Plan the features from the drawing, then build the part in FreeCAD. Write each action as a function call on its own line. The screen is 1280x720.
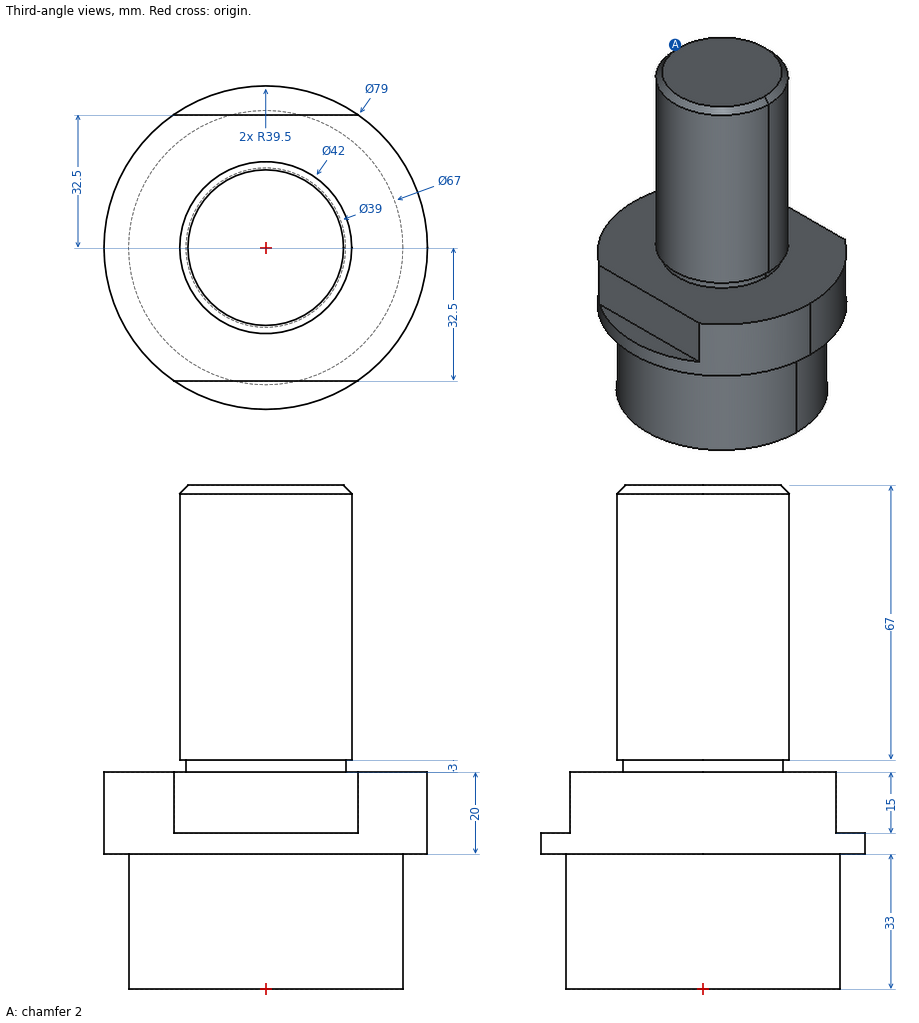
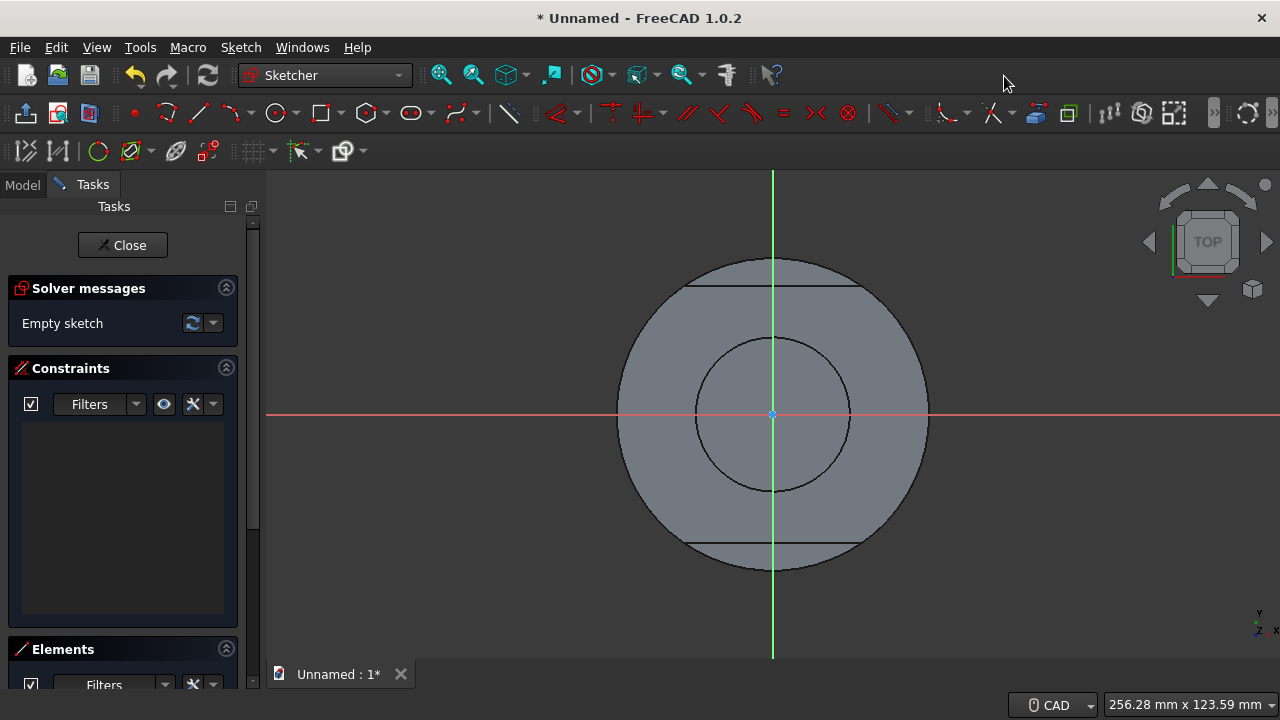
scroll(856, 415, up, 3)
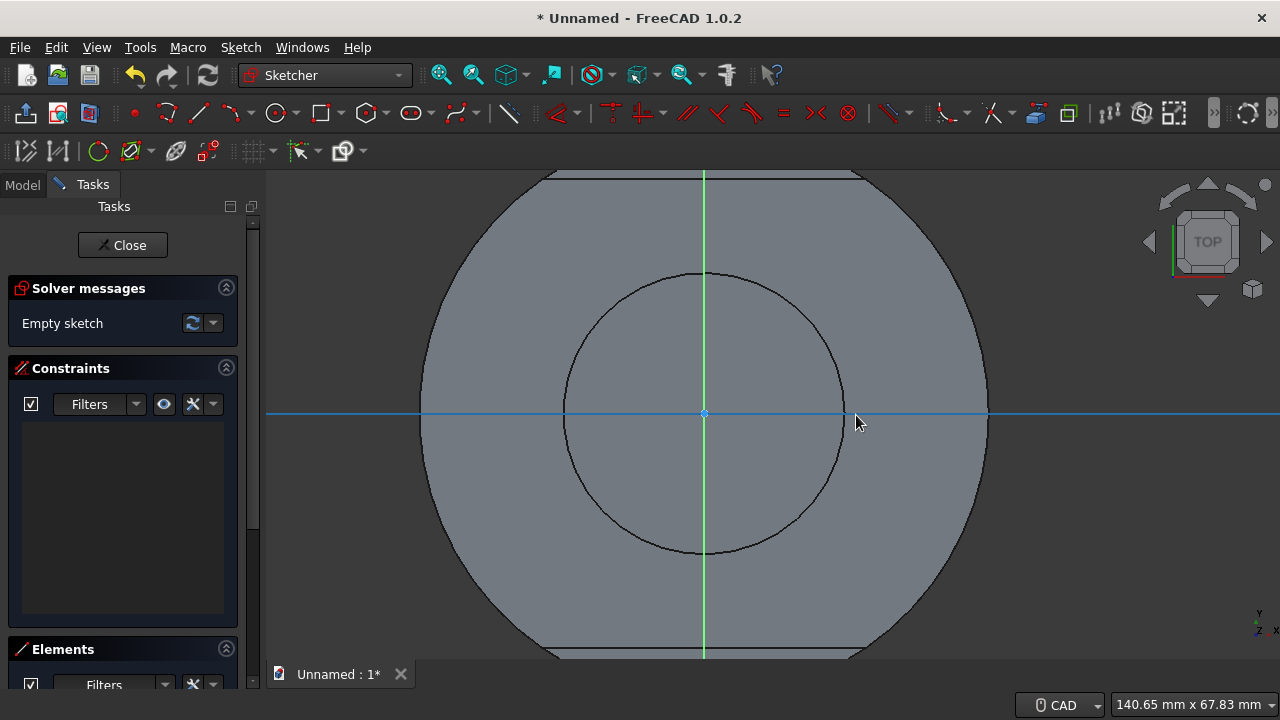
click(276, 114)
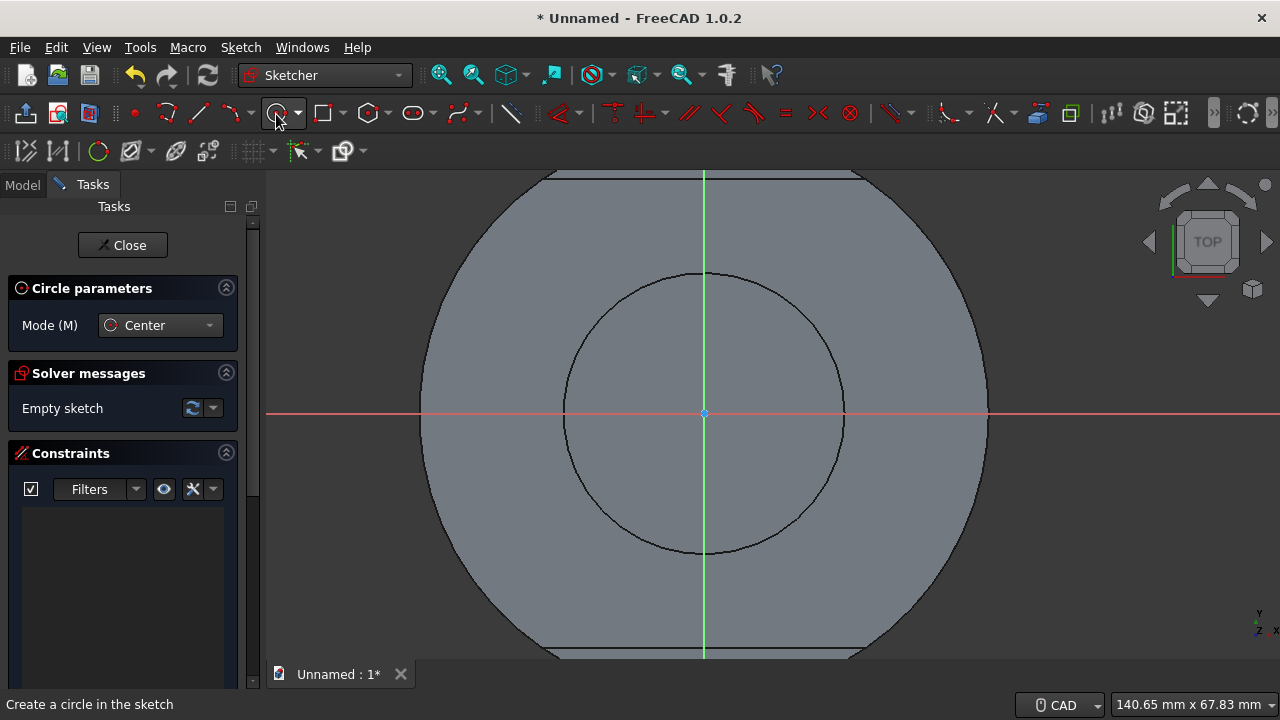
click(704, 414)
move(811, 307)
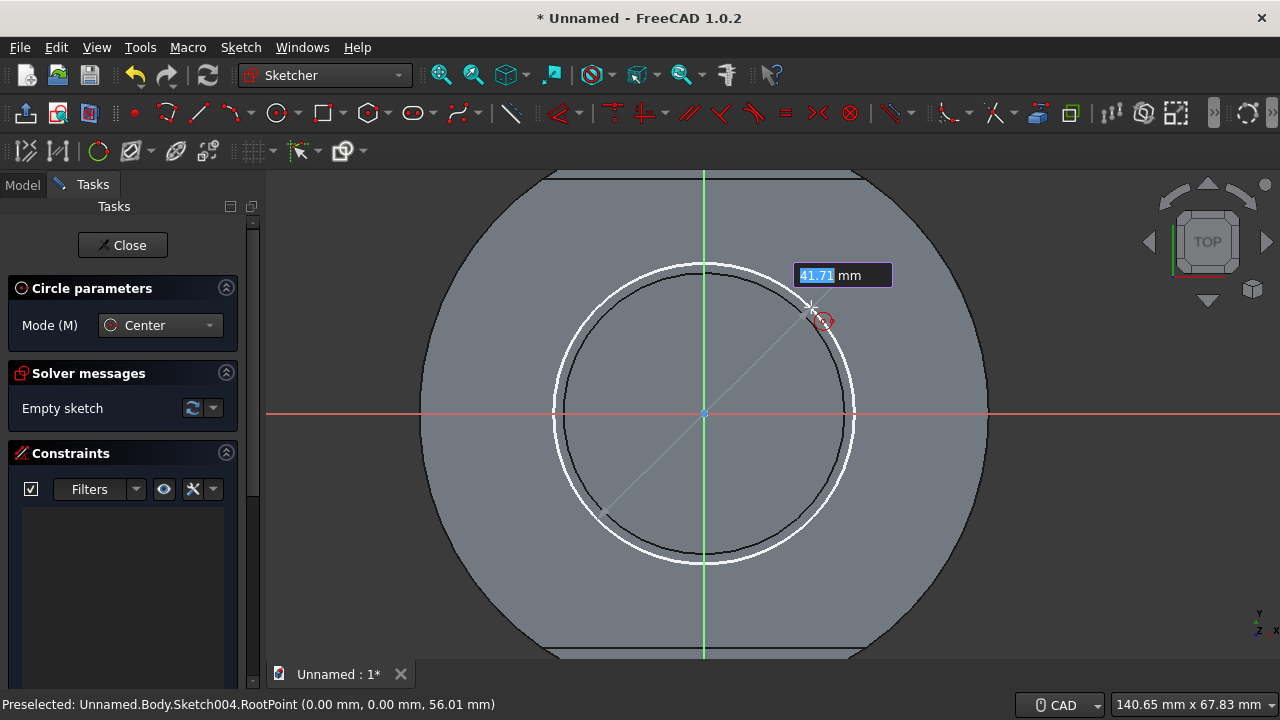
text(42)
key(Return)
key(Escape)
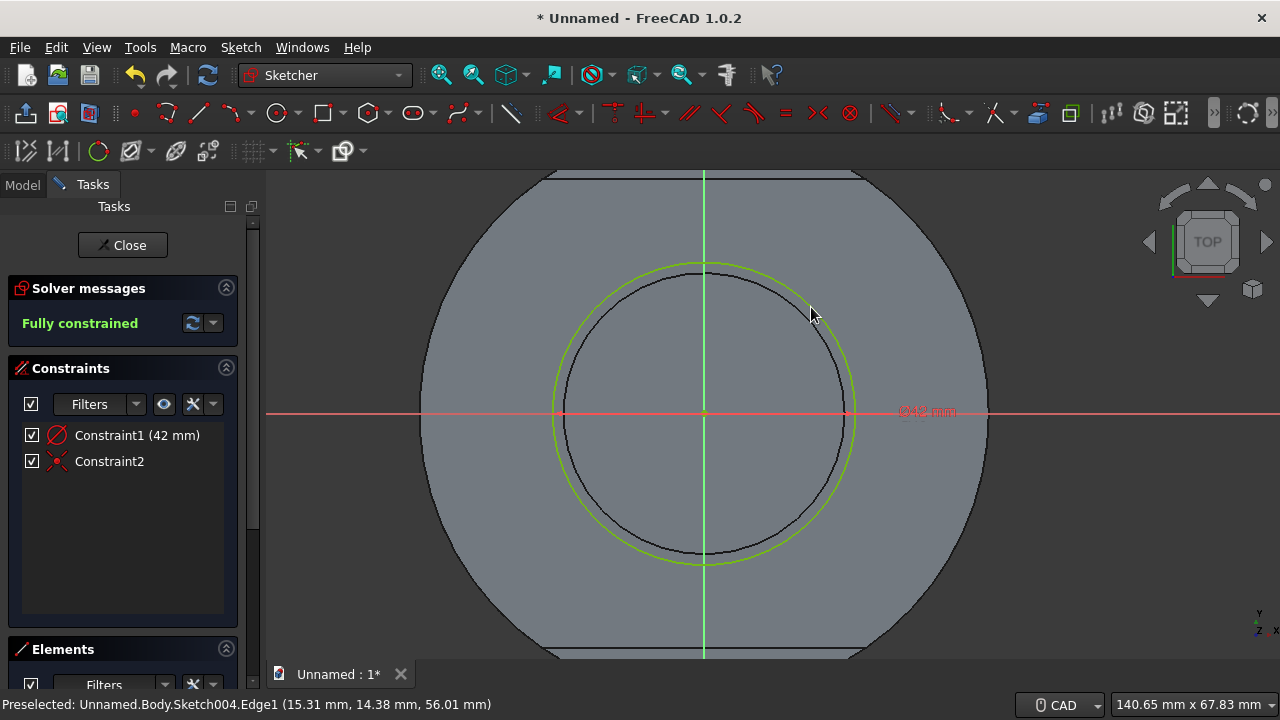
click(123, 245)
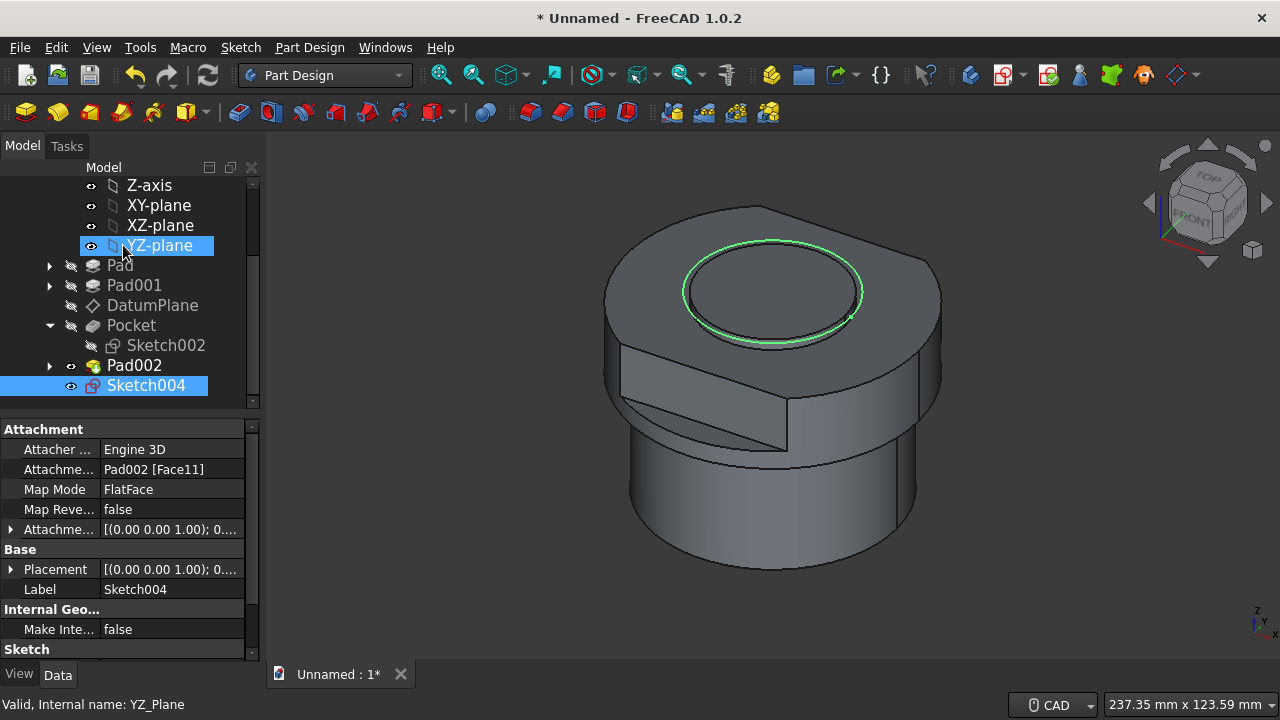
click(26, 112)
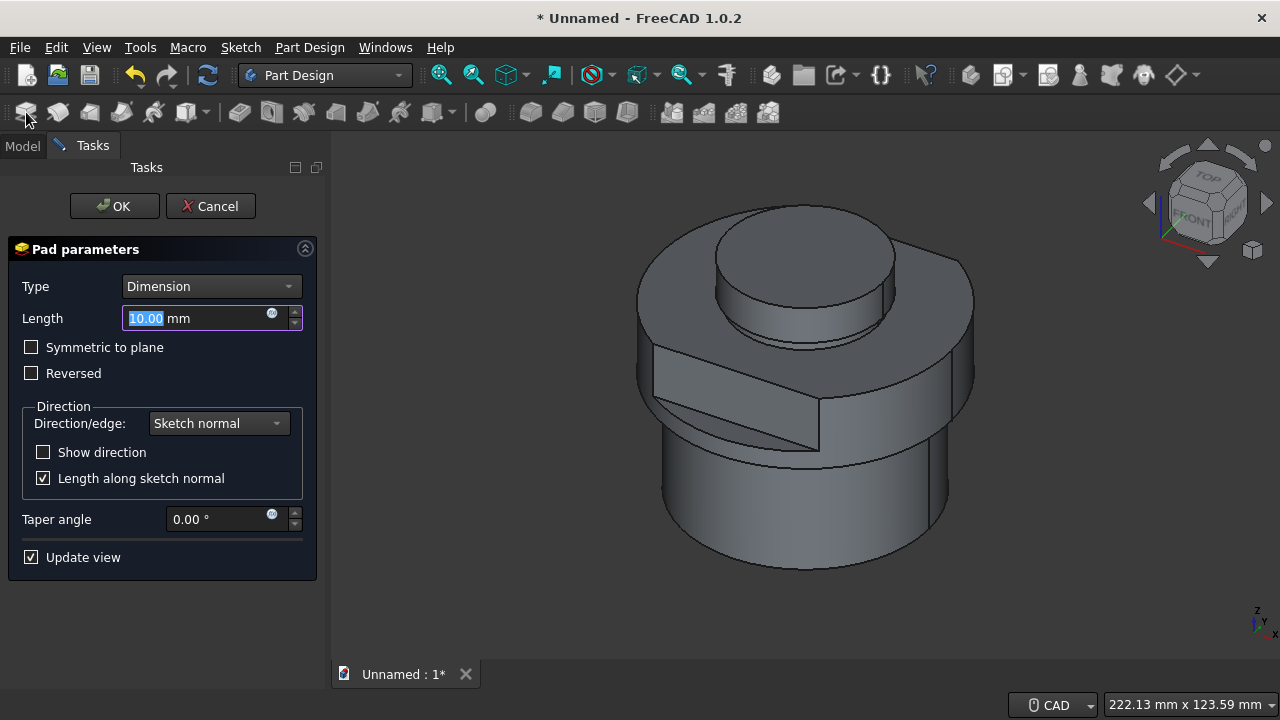
text(67)
key(Tab)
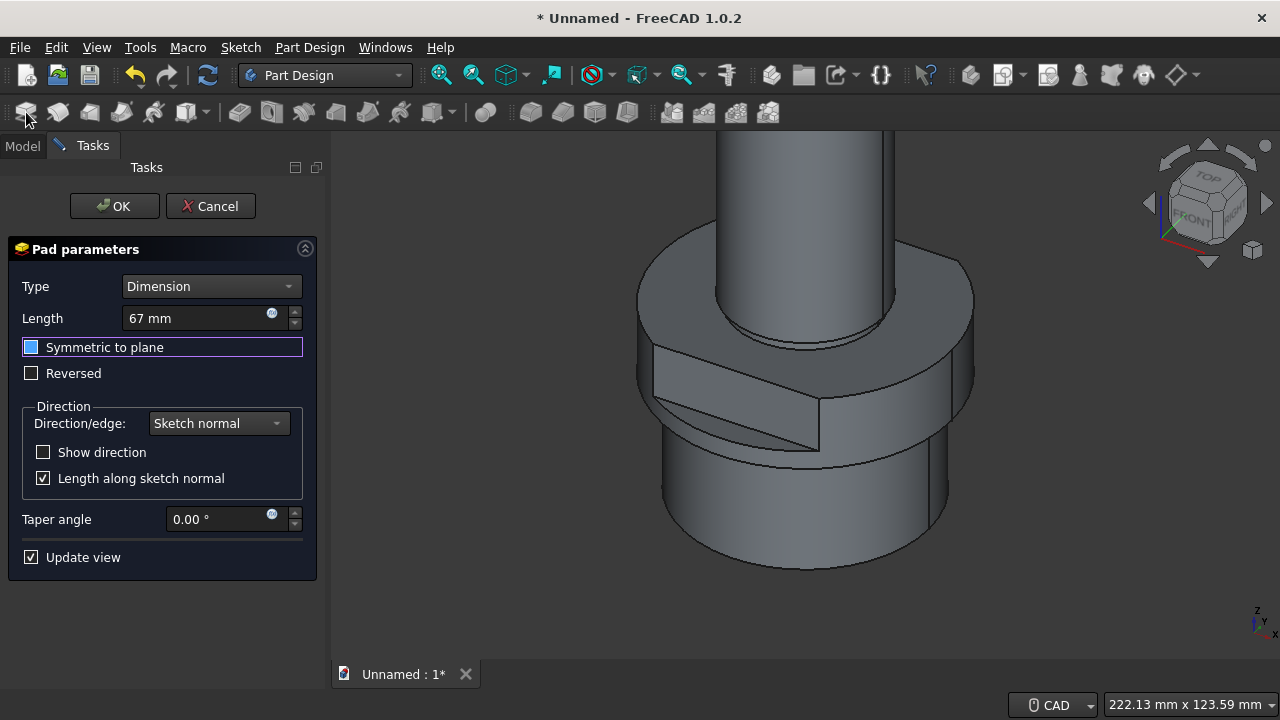
click(115, 206)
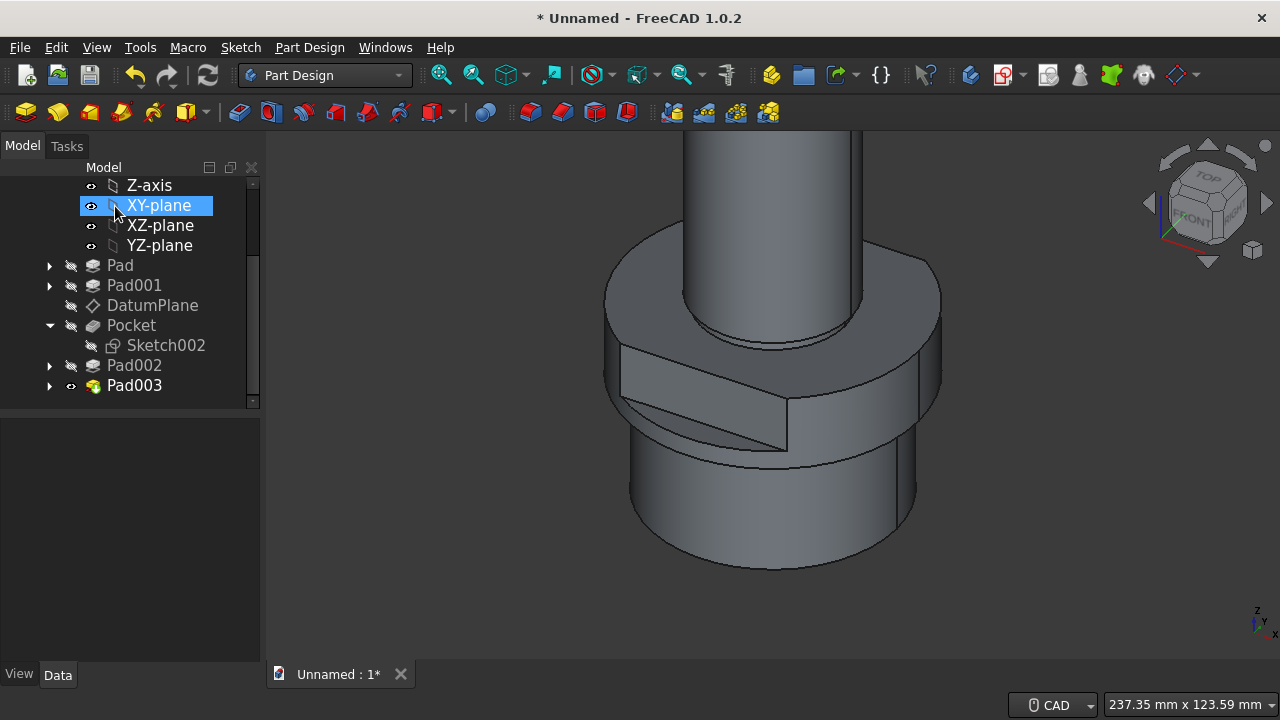
click(442, 76)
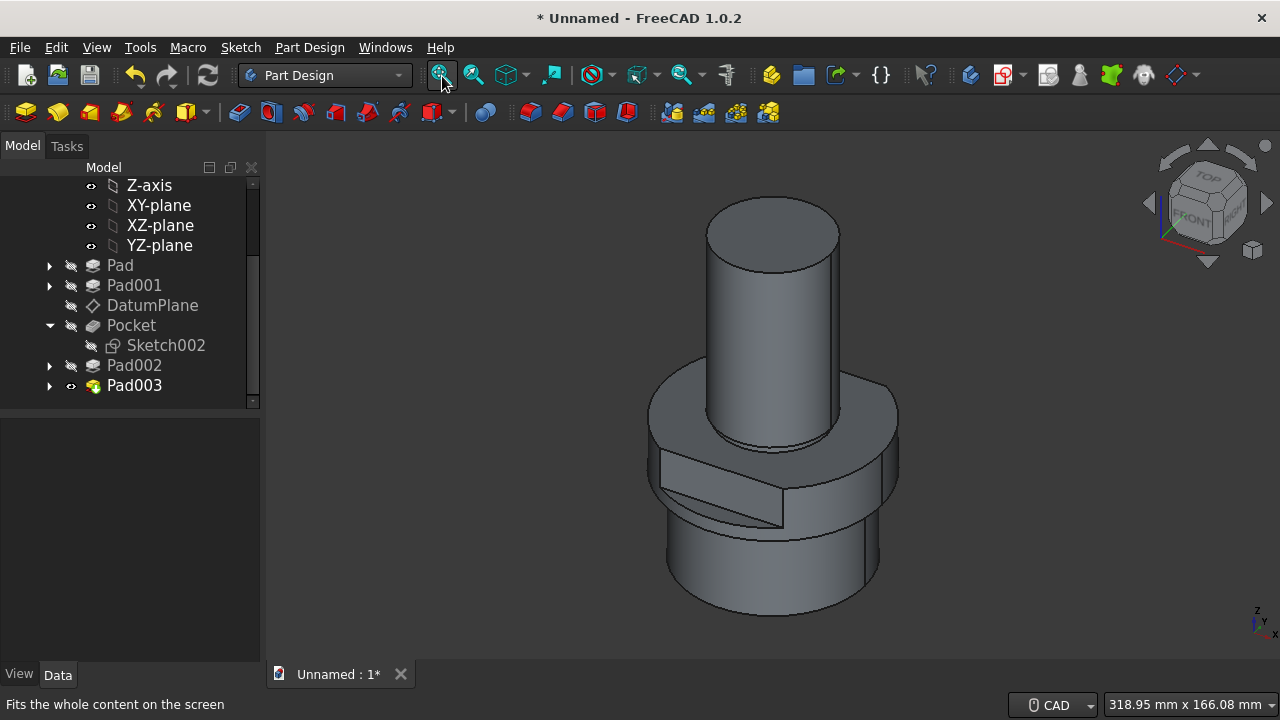
click(707, 238)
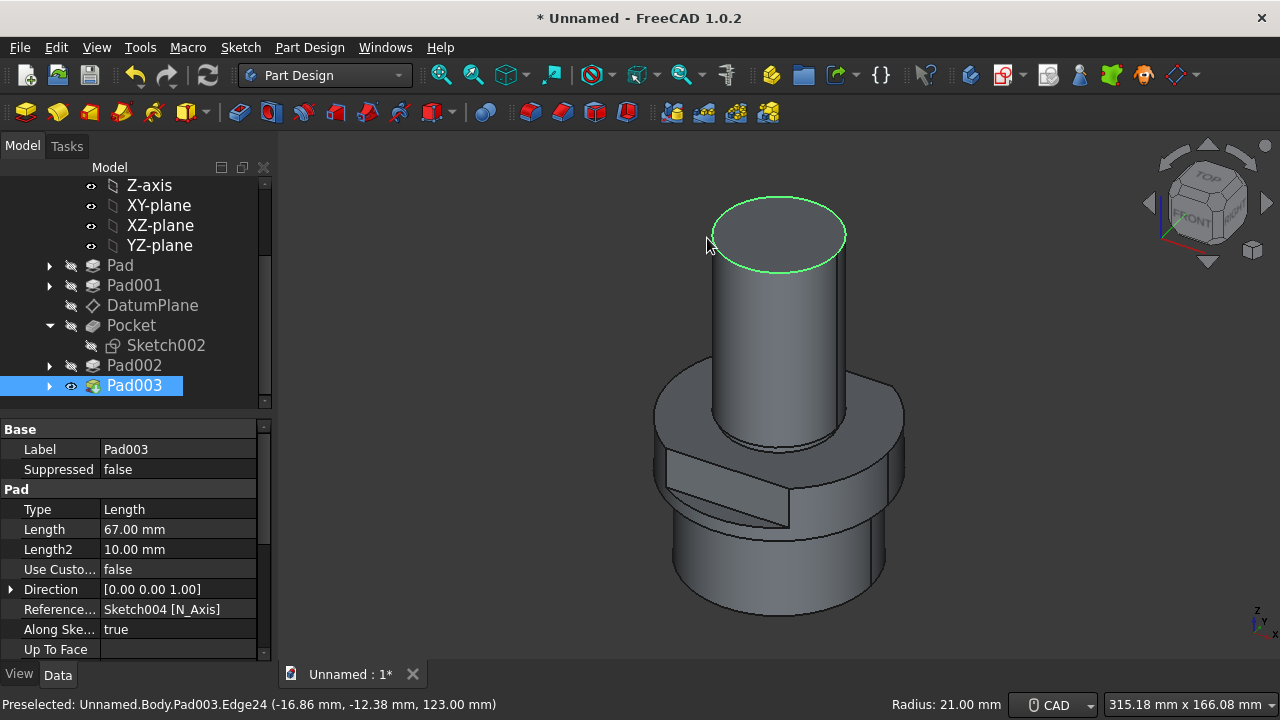
click(564, 112)